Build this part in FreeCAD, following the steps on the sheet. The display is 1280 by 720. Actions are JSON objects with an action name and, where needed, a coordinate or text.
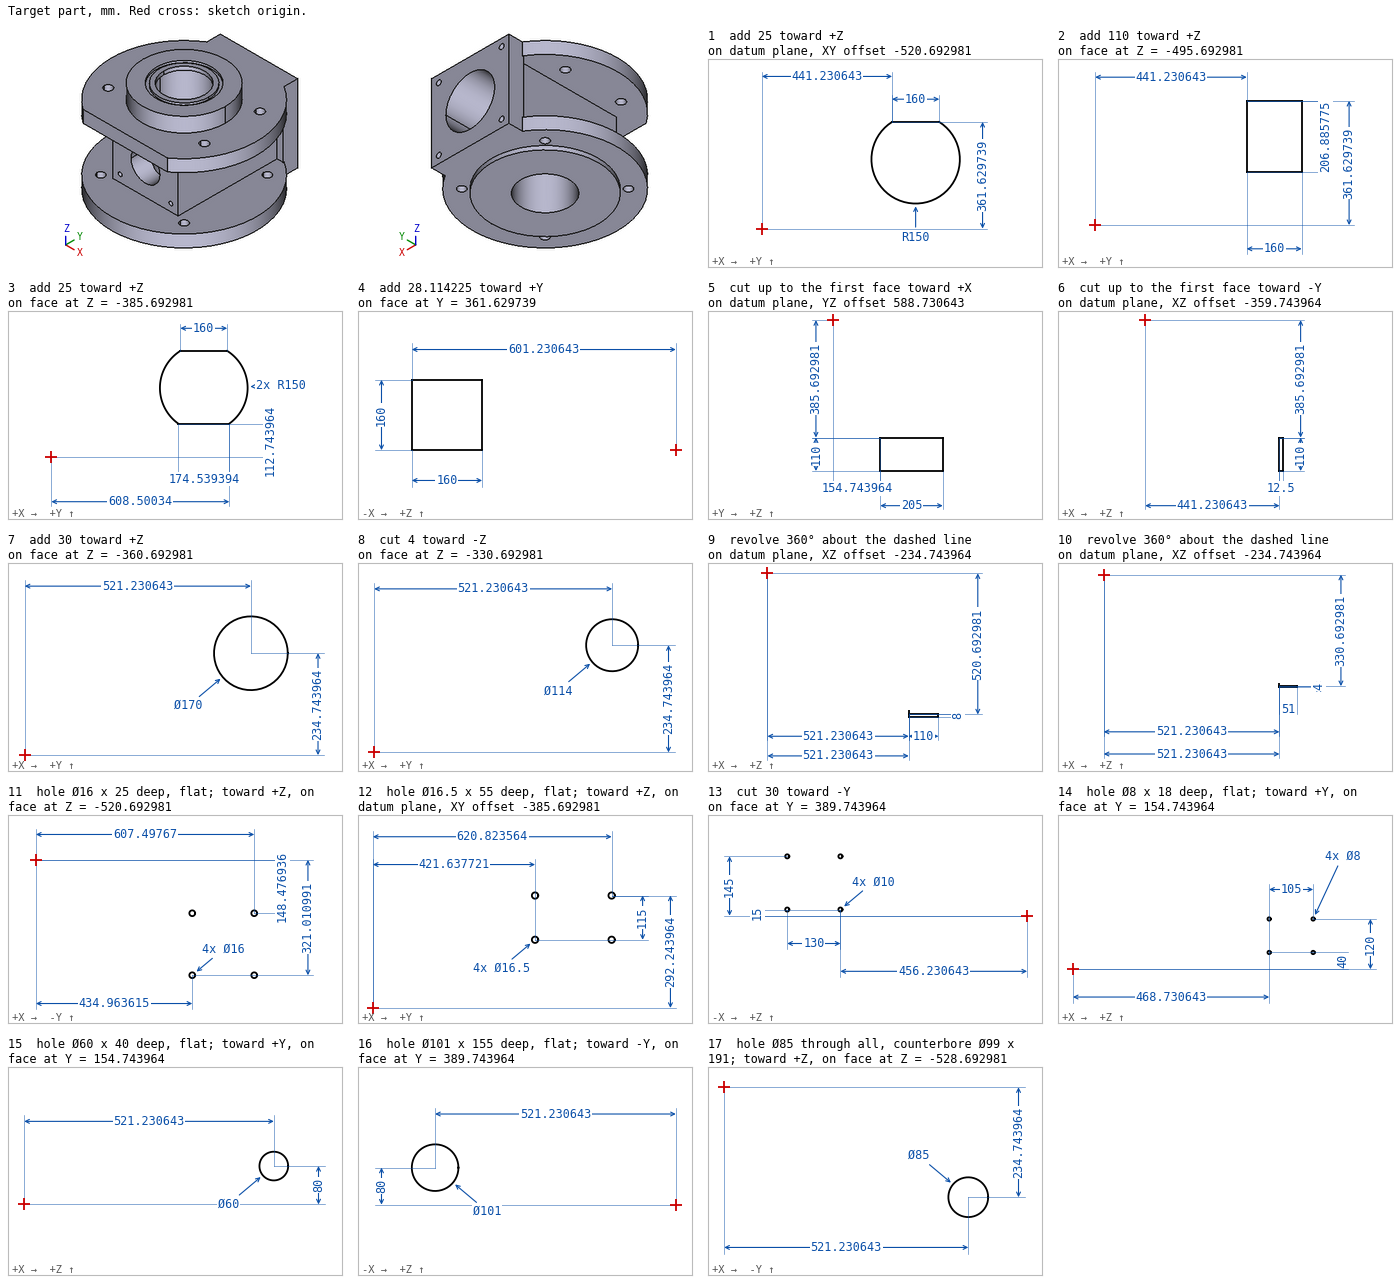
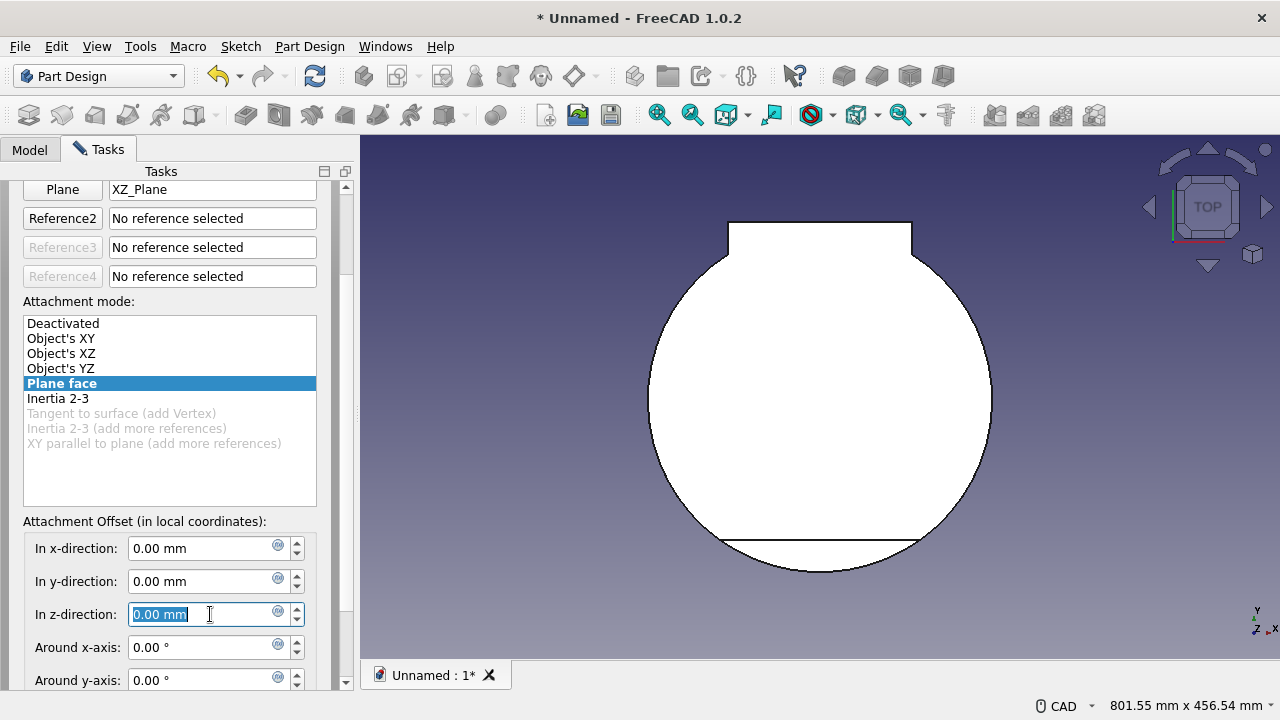
{"action": "type", "text": "-359.743964"}
{"action": "key", "text": "Tab"}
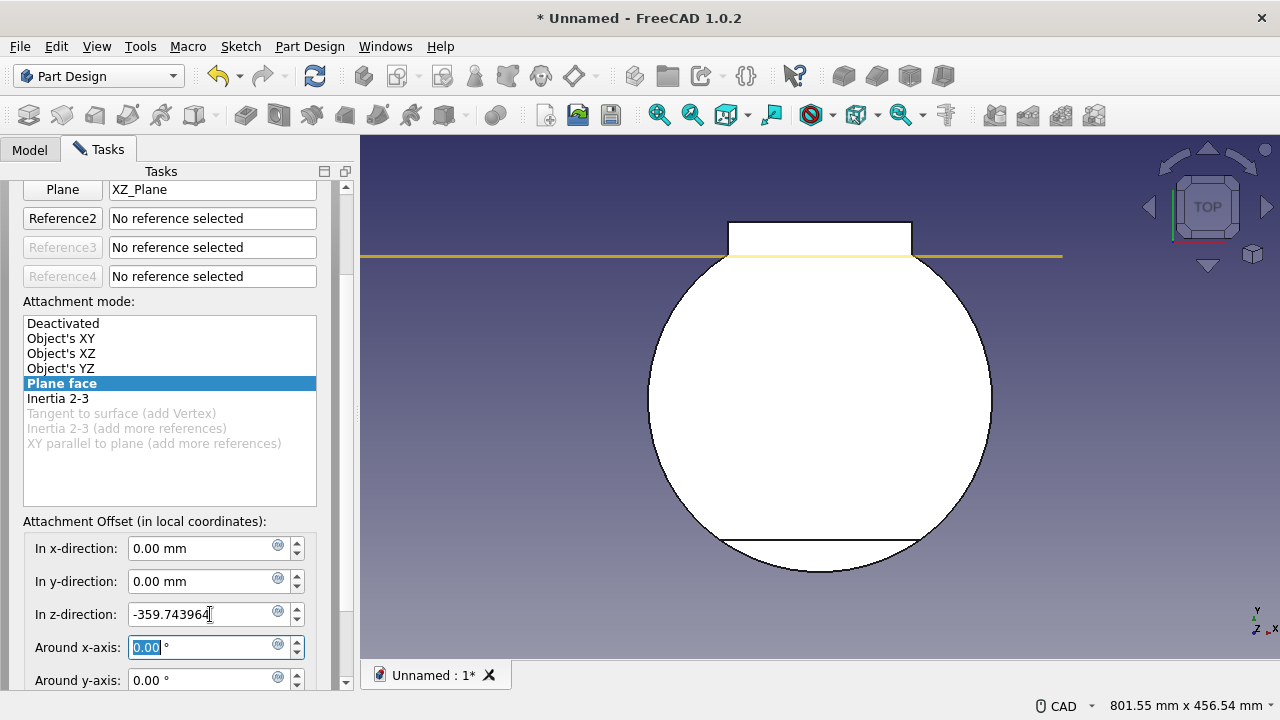
{"action": "scroll", "coordinate": [346, 436], "scroll_direction": "up", "scroll_amount": 3}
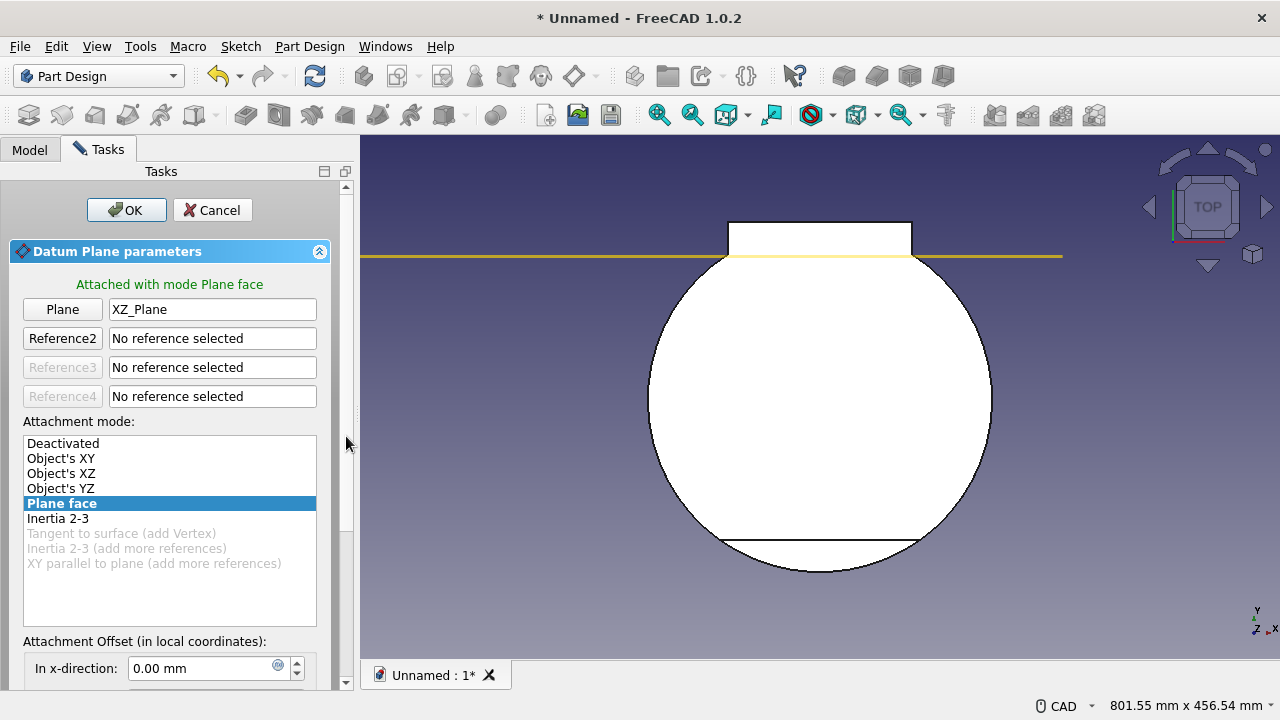
{"action": "left_click", "coordinate": [127, 210]}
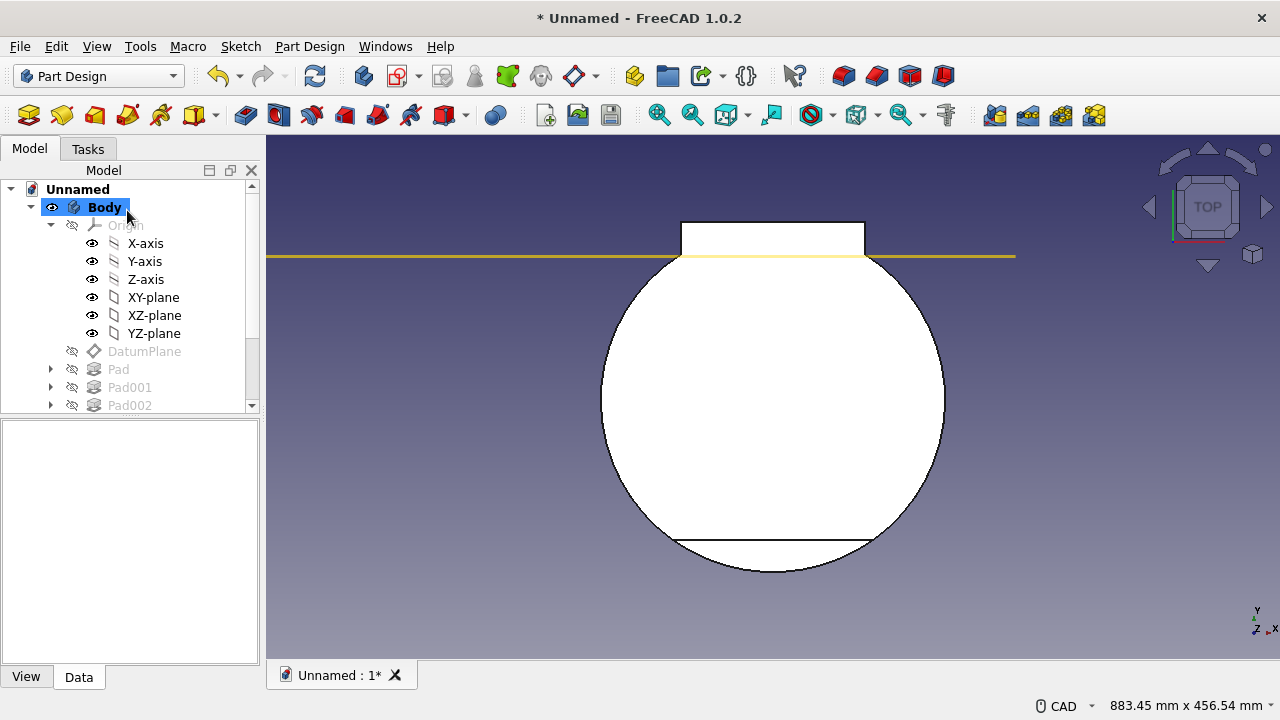
{"action": "scroll", "coordinate": [101, 293], "scroll_direction": "down", "scroll_amount": 3}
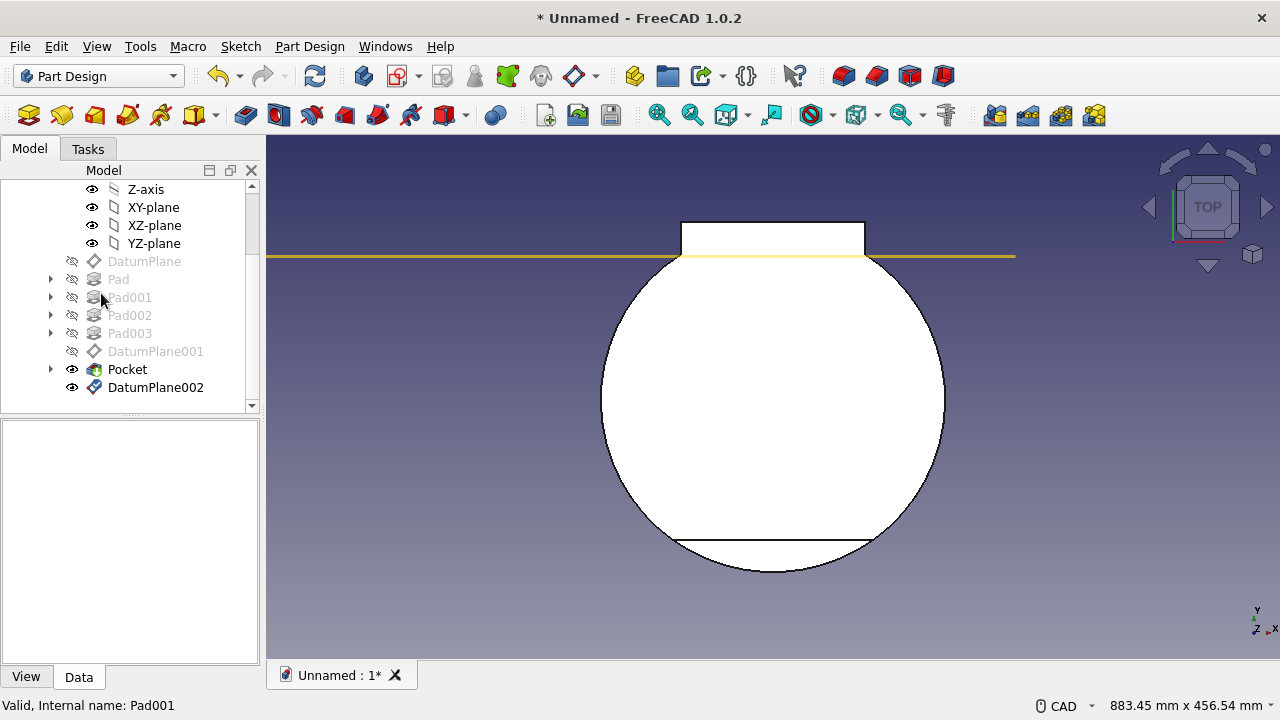
{"action": "left_click", "coordinate": [117, 387]}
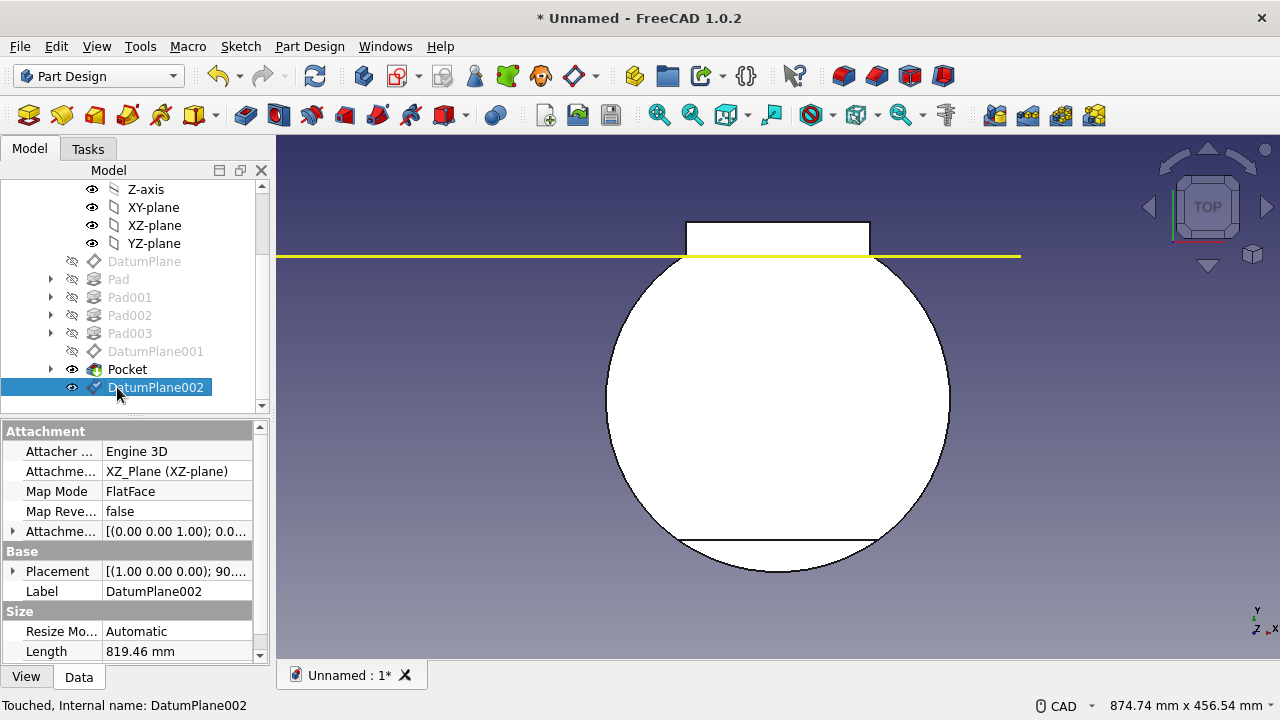
{"action": "left_click", "coordinate": [396, 76]}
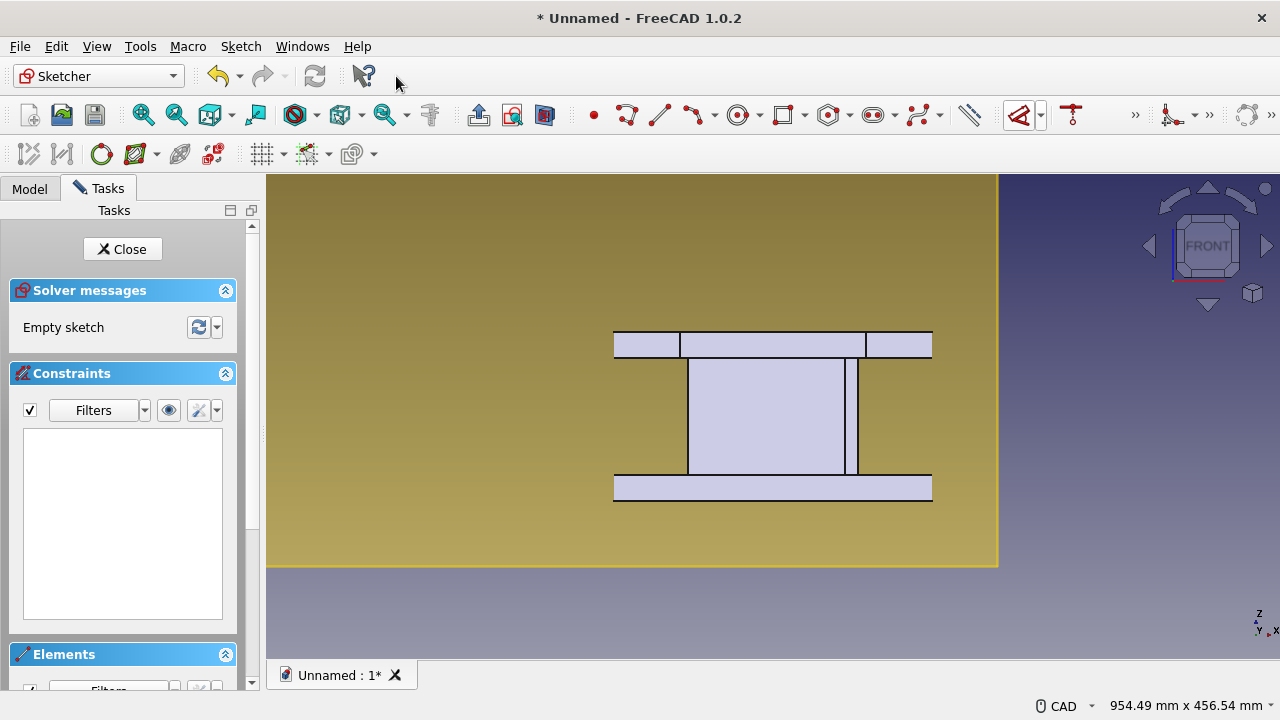
{"action": "left_click", "coordinate": [545, 116]}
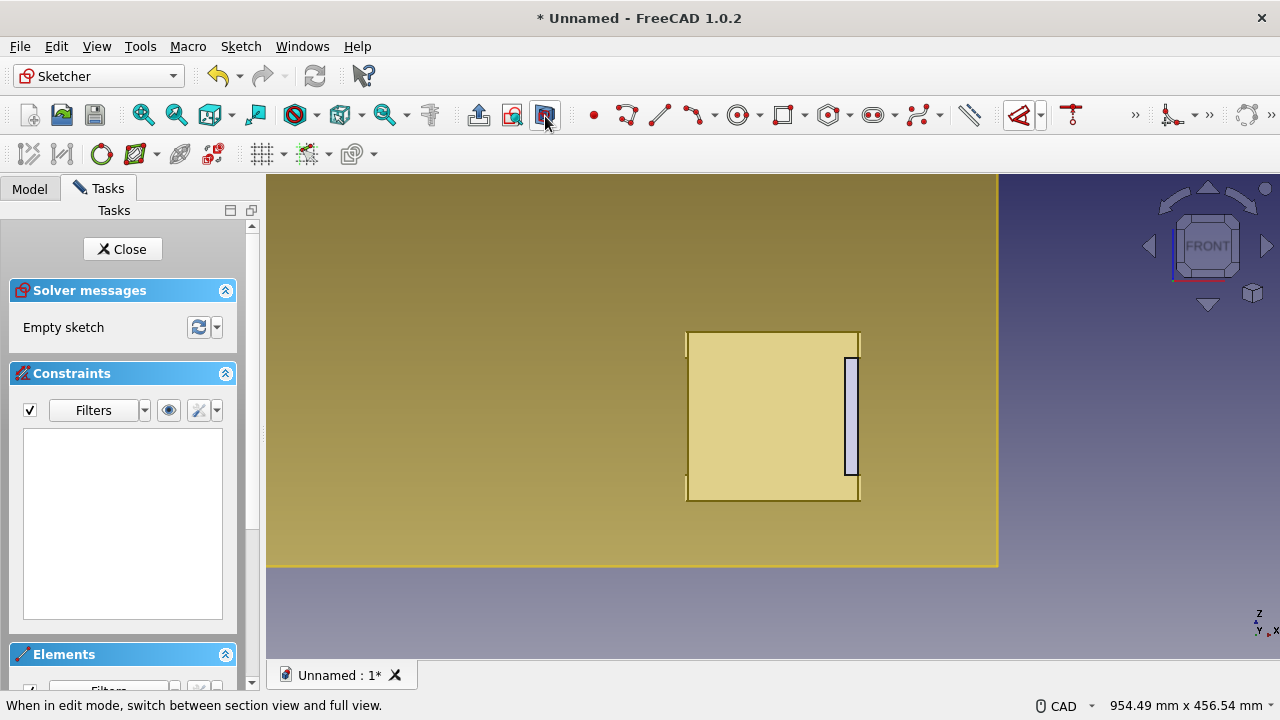
{"action": "scroll", "coordinate": [689, 416], "scroll_direction": "up", "scroll_amount": 5}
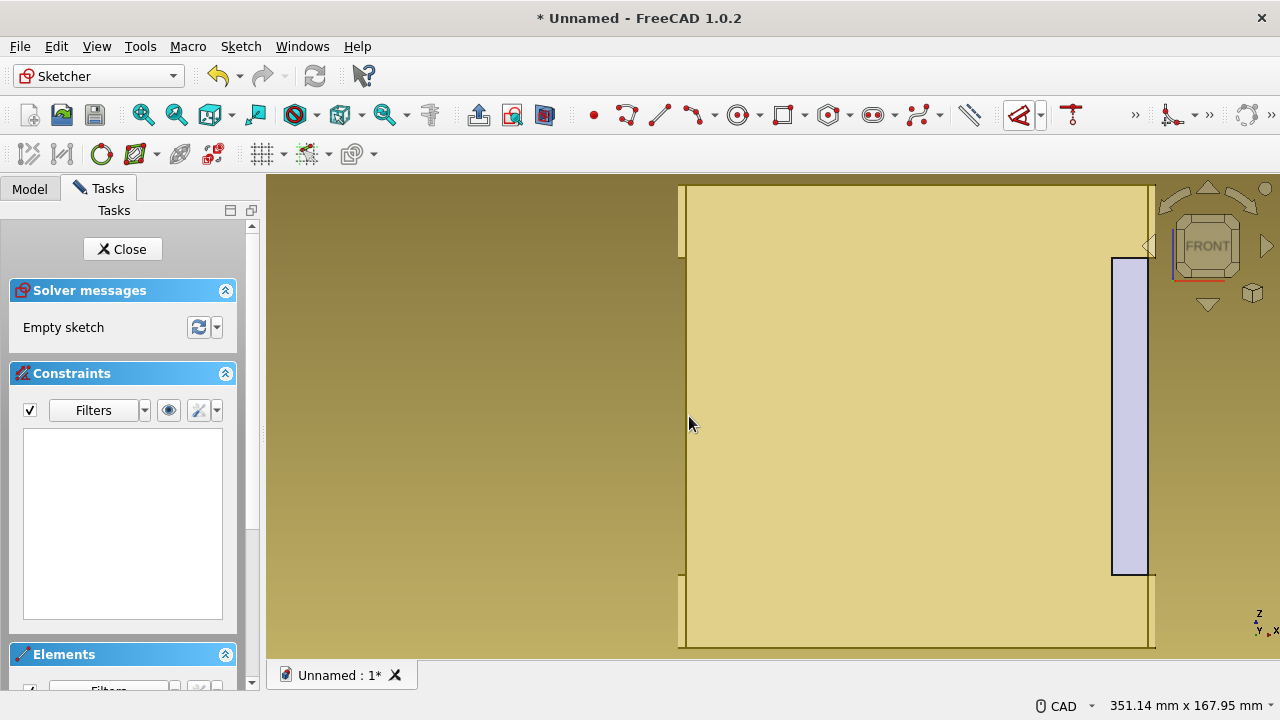
{"action": "left_click", "coordinate": [782, 116]}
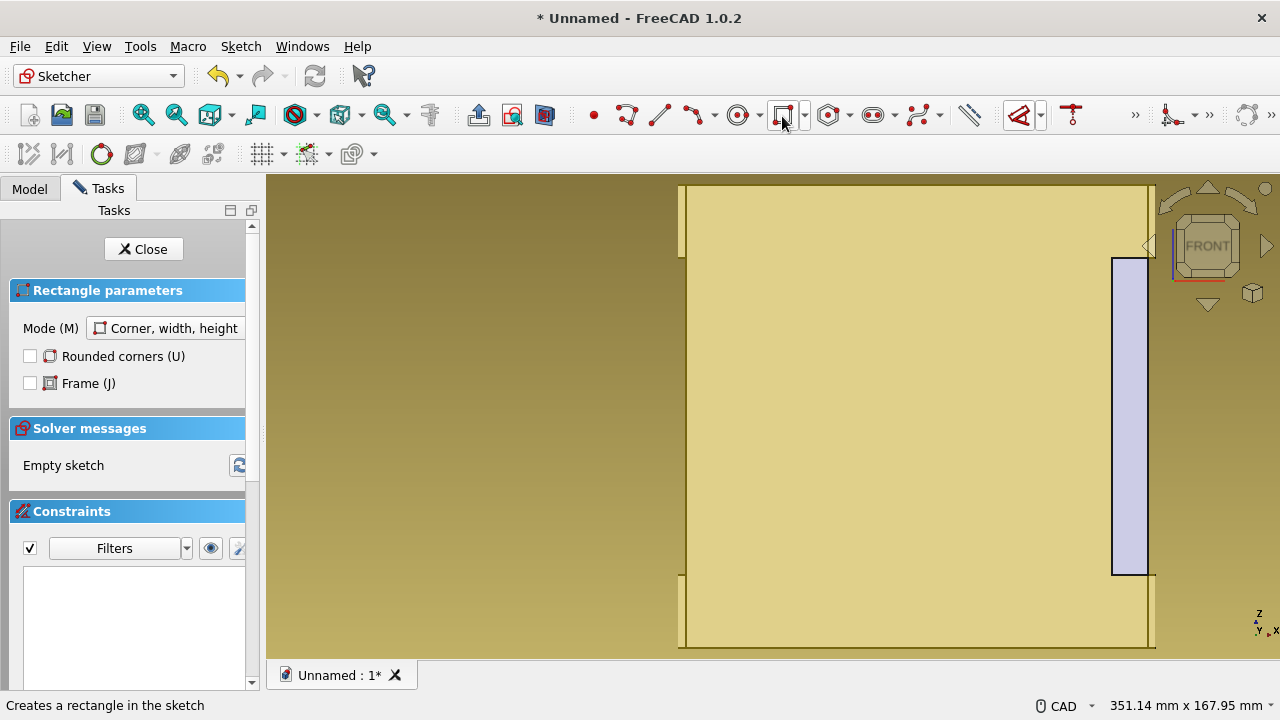
{"action": "left_click", "coordinate": [686, 258]}
{"action": "left_click", "coordinate": [722, 575]}
{"action": "key", "text": "Escape"}